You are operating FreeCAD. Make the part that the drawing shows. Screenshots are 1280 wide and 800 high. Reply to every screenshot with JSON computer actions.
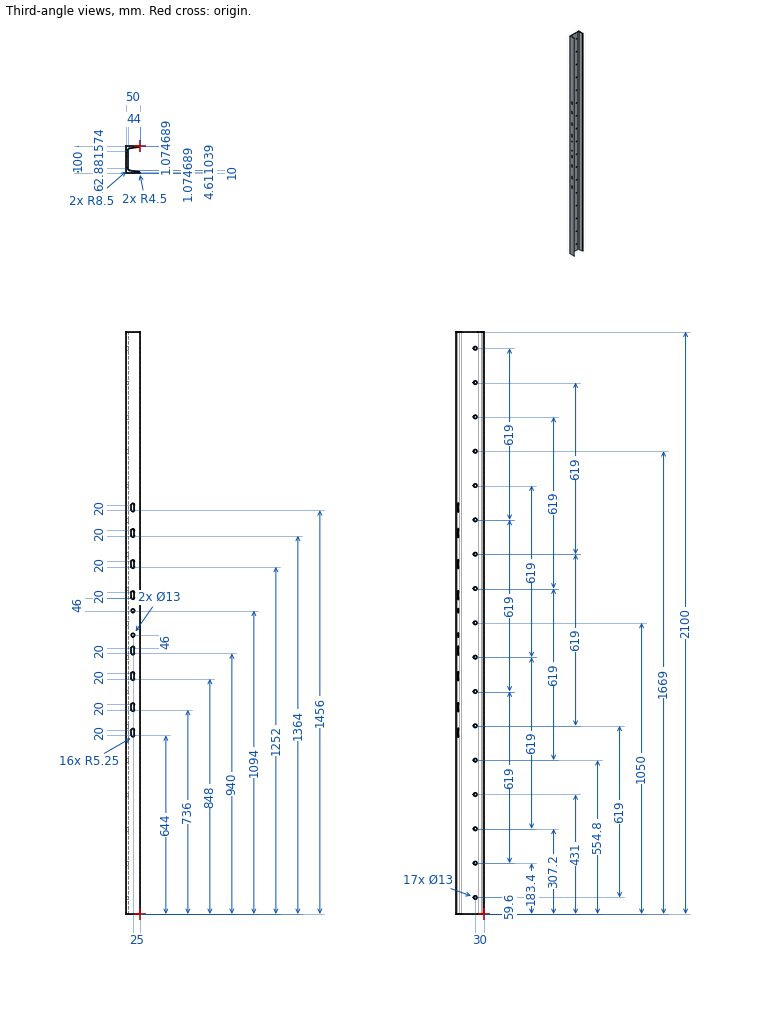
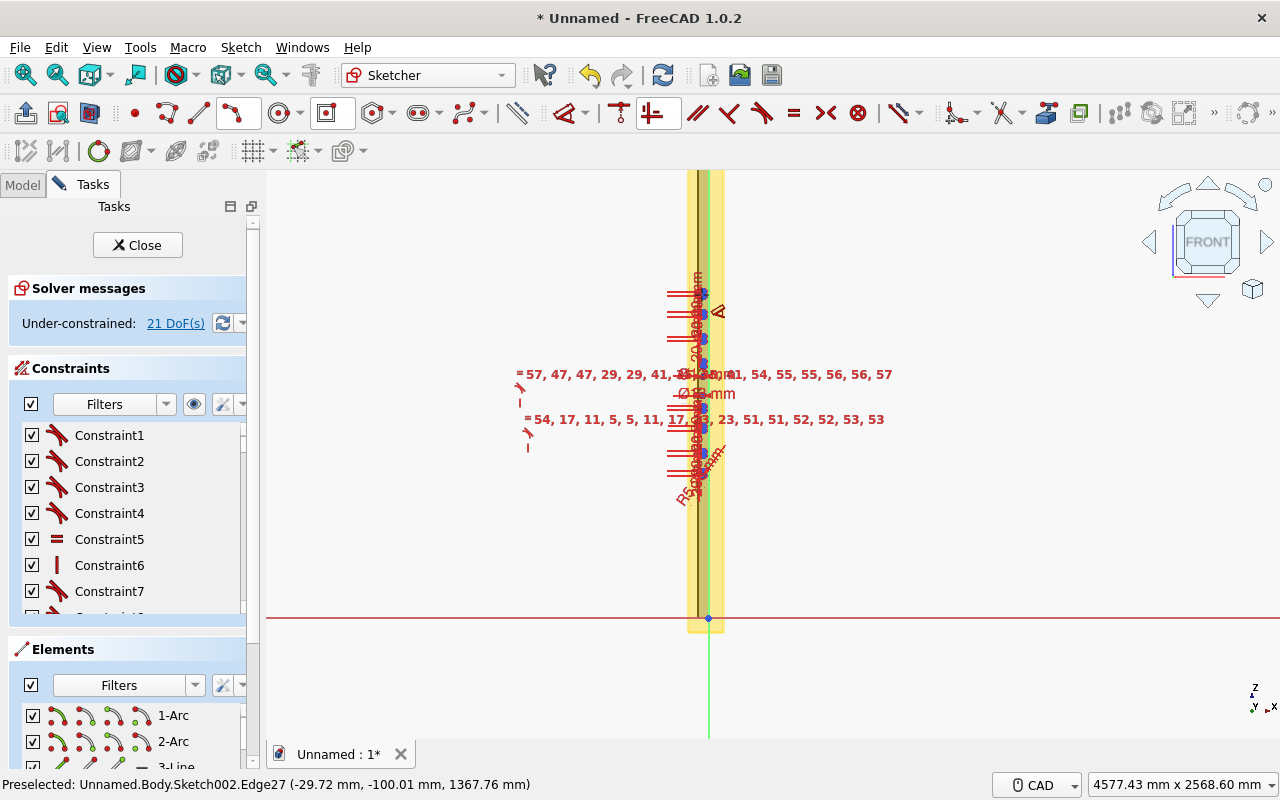
{"action": "scroll", "coordinate": [702, 365], "scroll_direction": "up", "scroll_amount": 12}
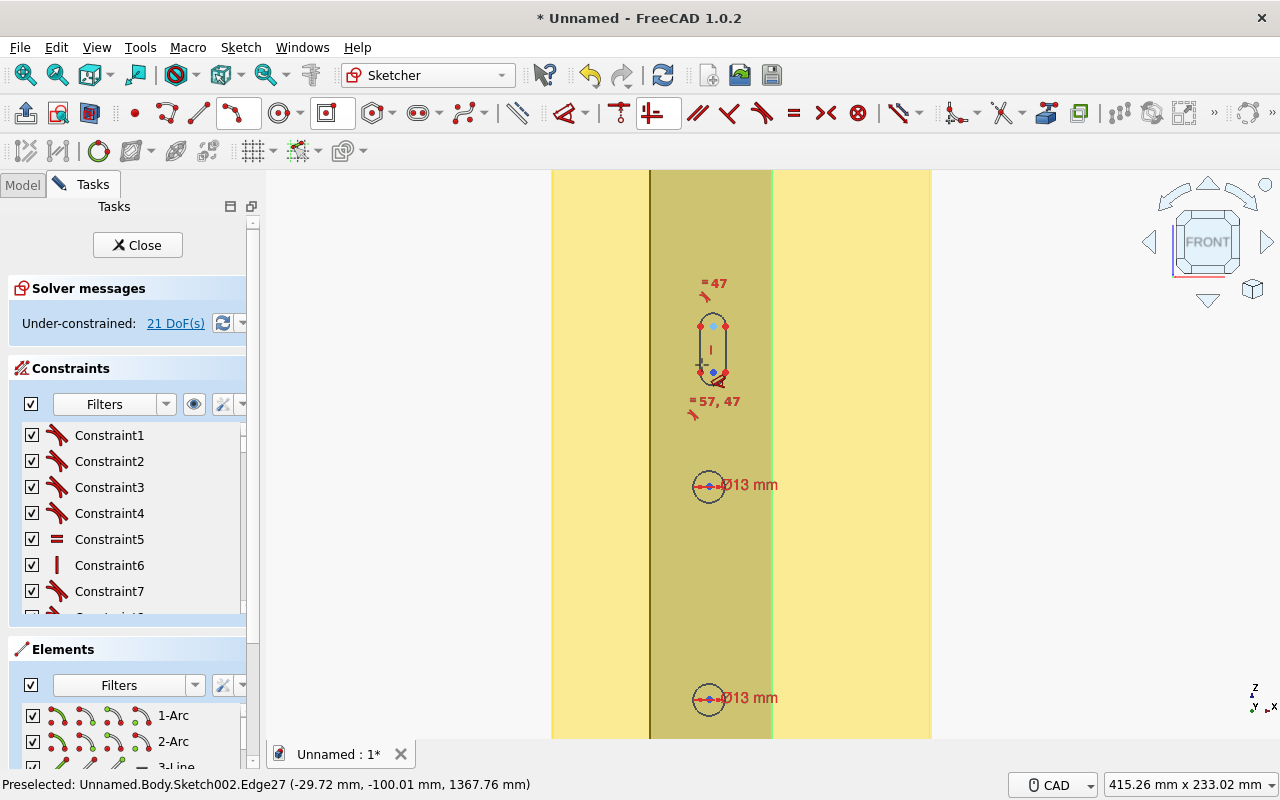
{"action": "left_click", "coordinate": [700, 359]}
{"action": "left_click", "coordinate": [666, 349]}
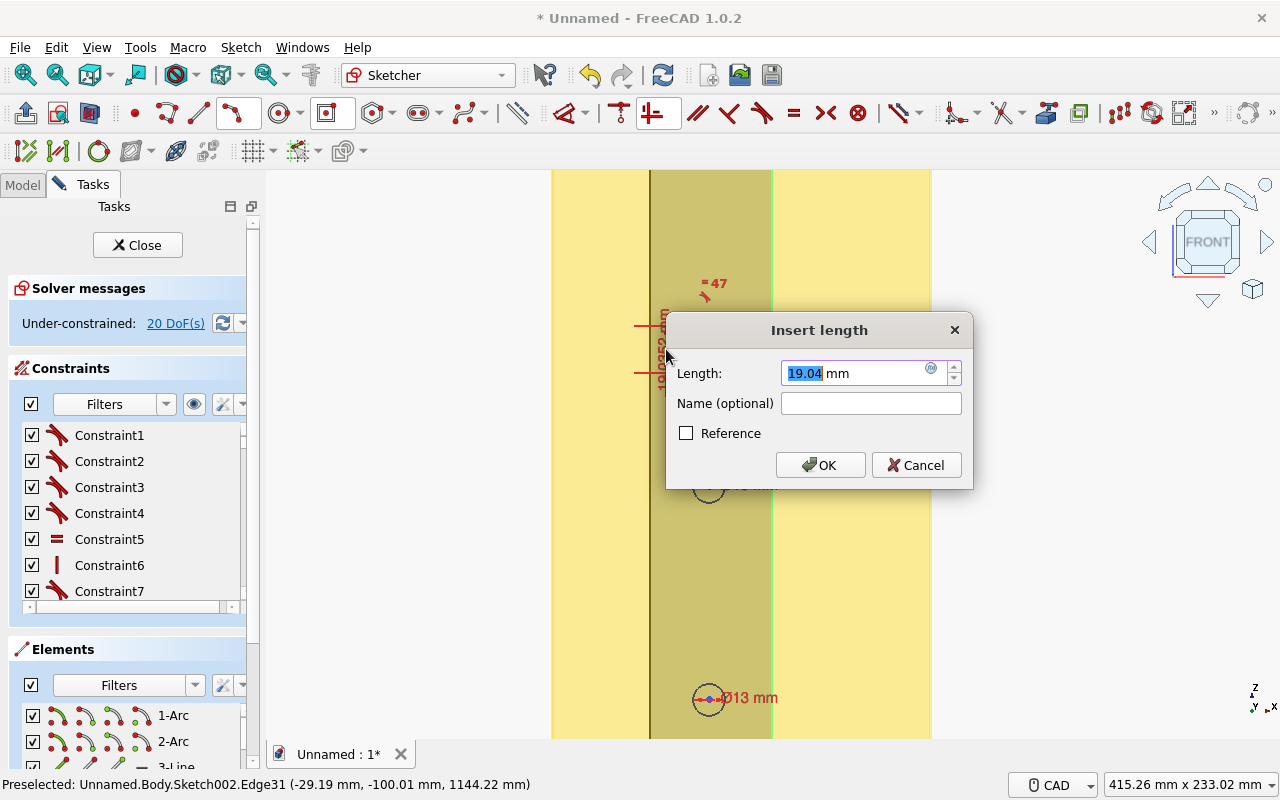
{"action": "type", "text": "20"}
{"action": "key", "text": "Return"}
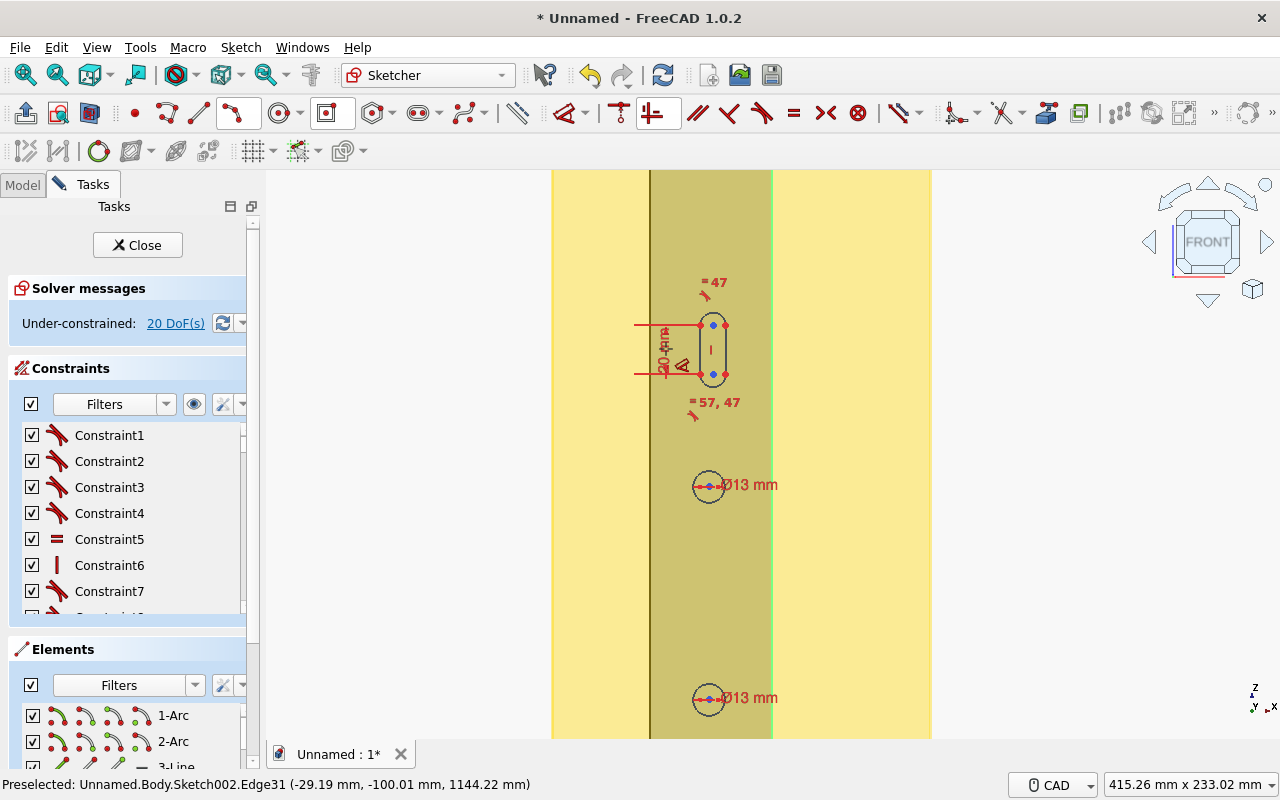
{"action": "left_click", "coordinate": [709, 700]}
{"action": "left_click", "coordinate": [740, 666]}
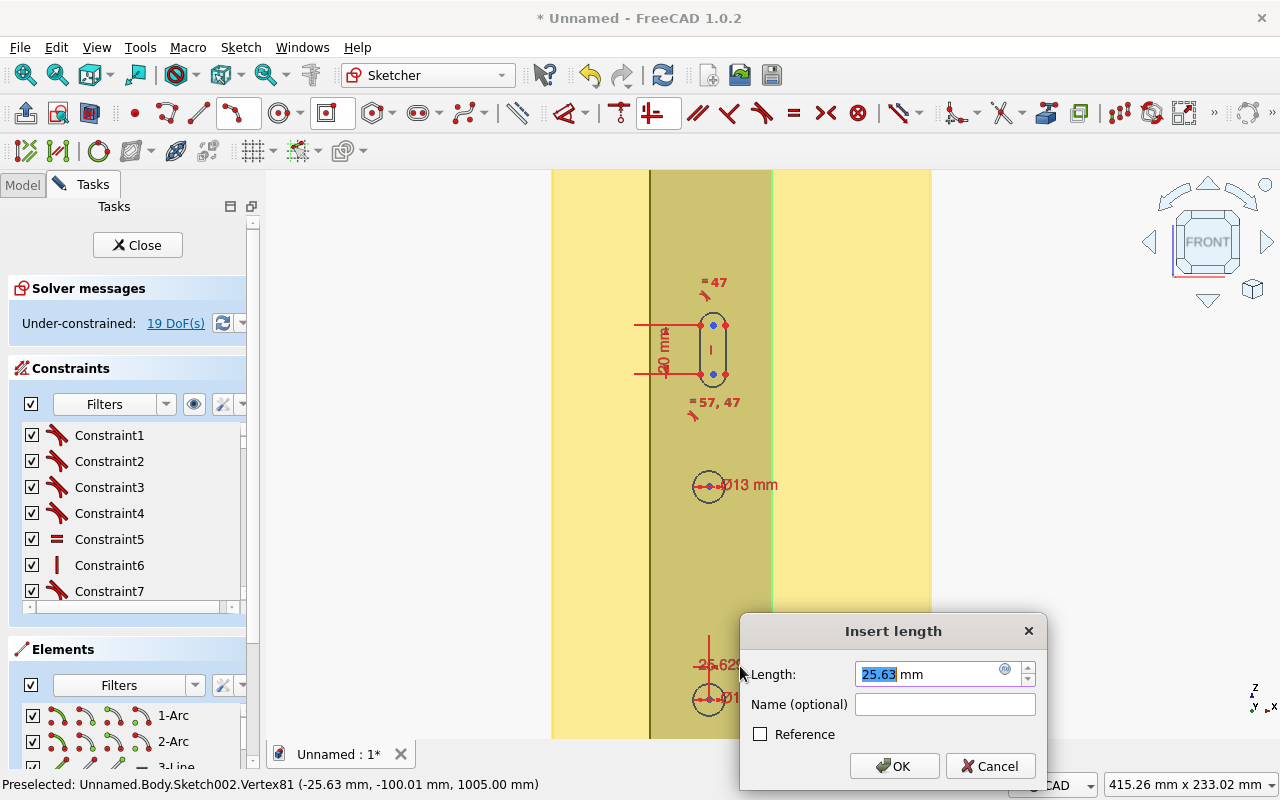
{"action": "type", "text": "25"}
{"action": "key", "text": "Return"}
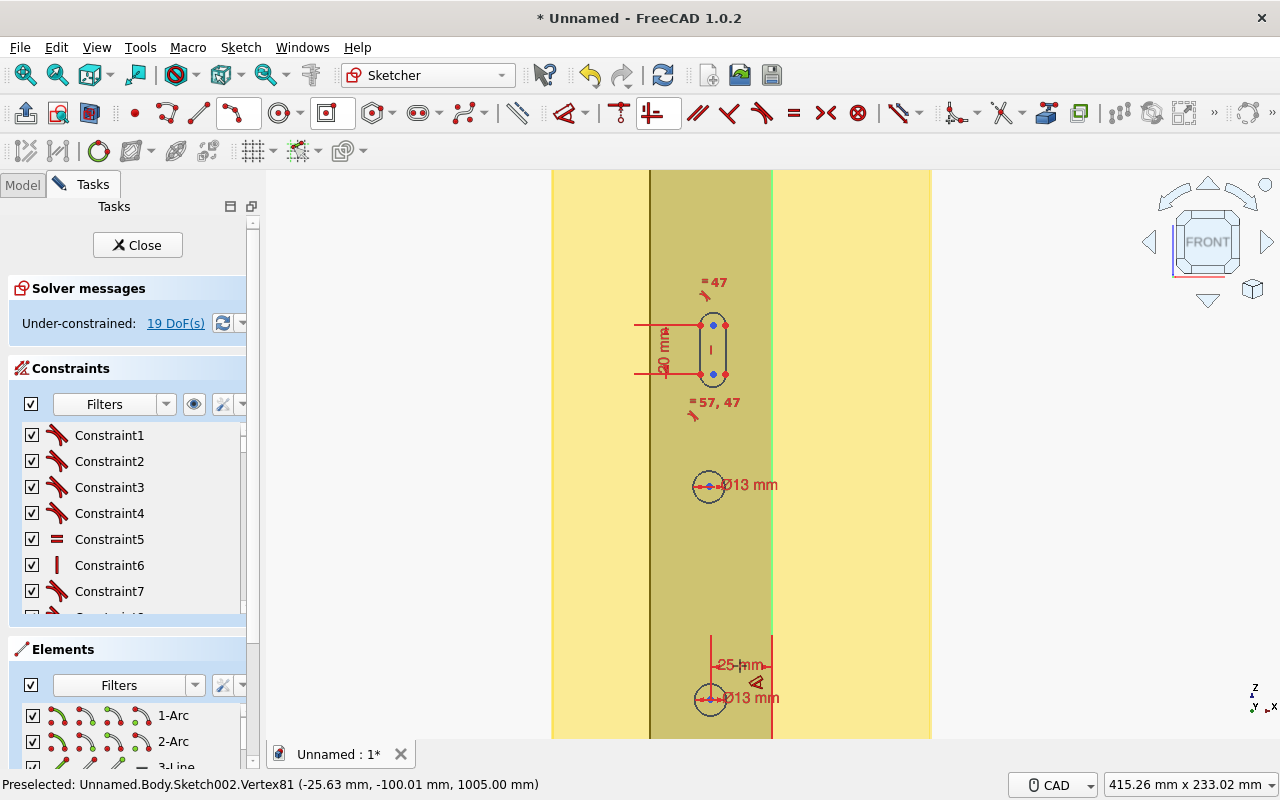
{"action": "left_click", "coordinate": [709, 487]}
{"action": "left_click", "coordinate": [740, 453]}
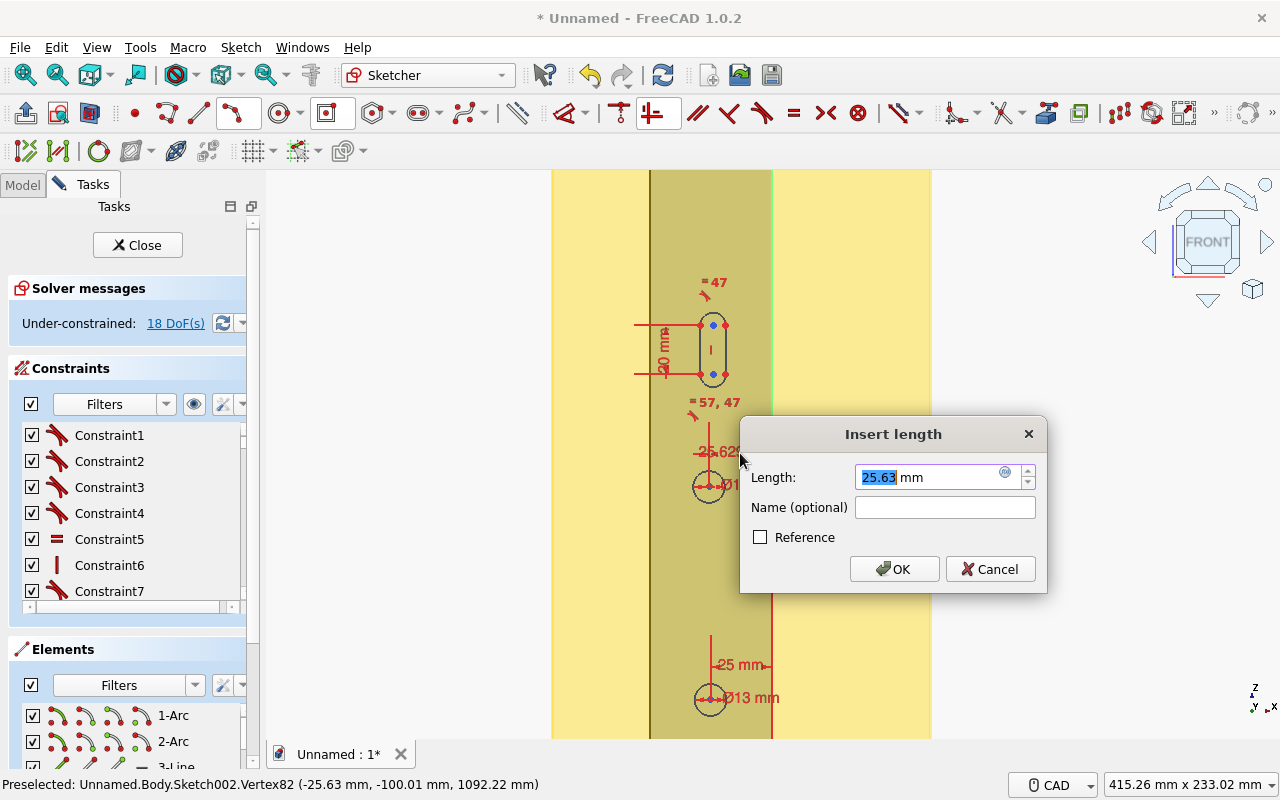
{"action": "type", "text": "25"}
{"action": "key", "text": "Return"}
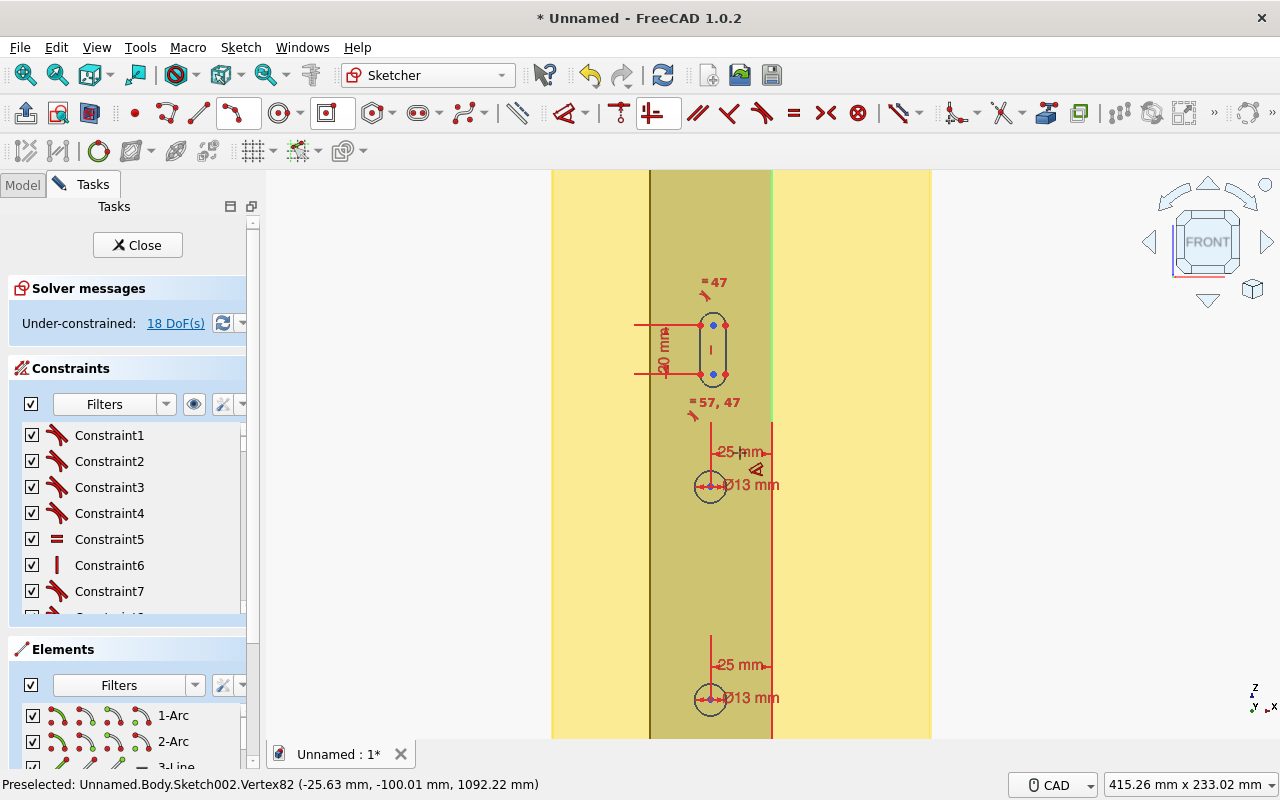
{"action": "scroll", "coordinate": [702, 366], "scroll_direction": "down", "scroll_amount": 12}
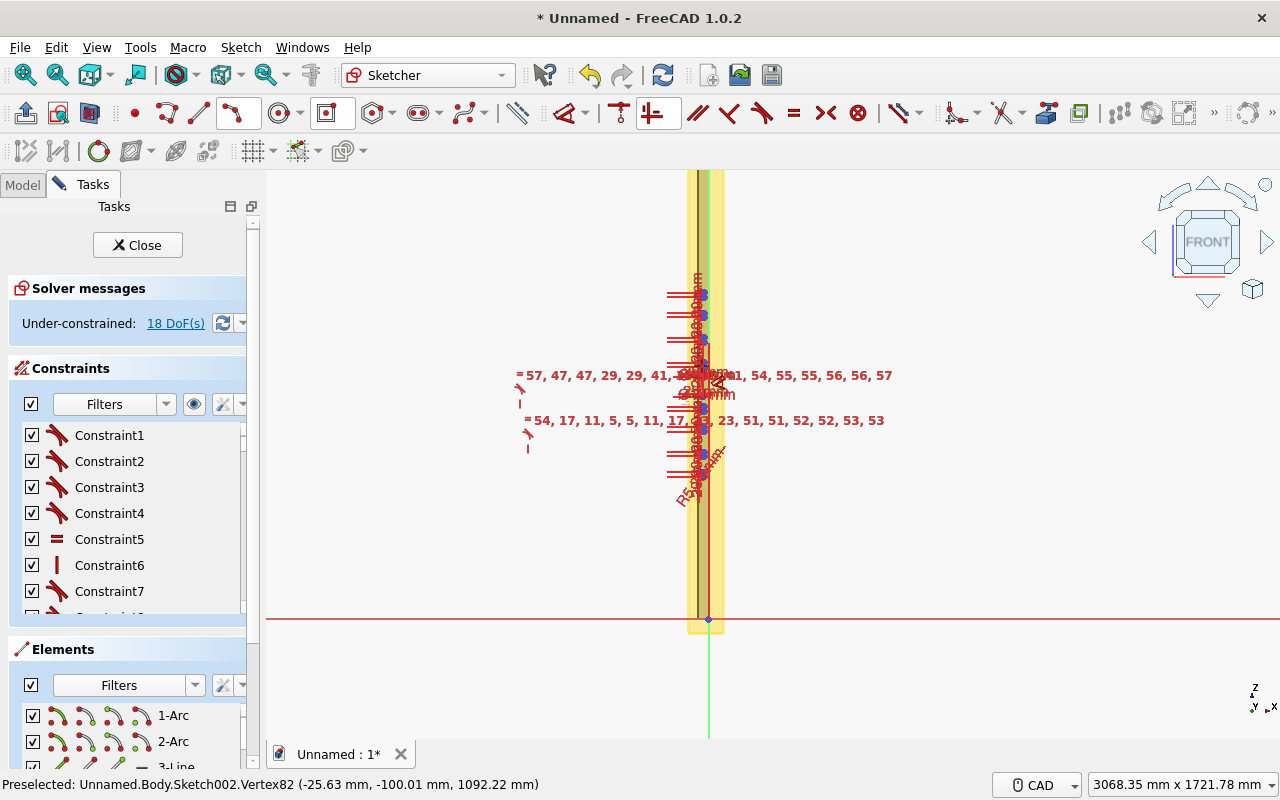
{"action": "scroll", "coordinate": [703, 477], "scroll_direction": "up", "scroll_amount": 12}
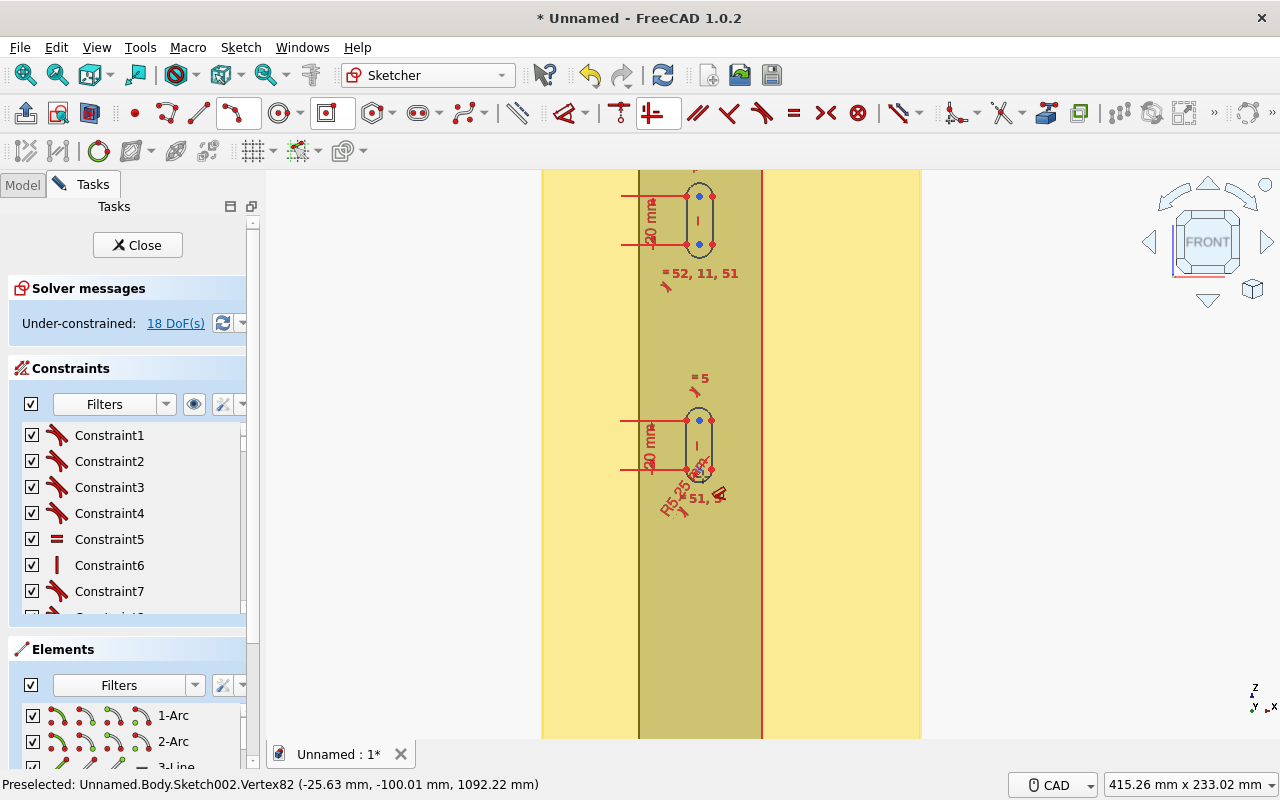
{"action": "left_click", "coordinate": [699, 470]}
{"action": "left_click", "coordinate": [730, 436]}